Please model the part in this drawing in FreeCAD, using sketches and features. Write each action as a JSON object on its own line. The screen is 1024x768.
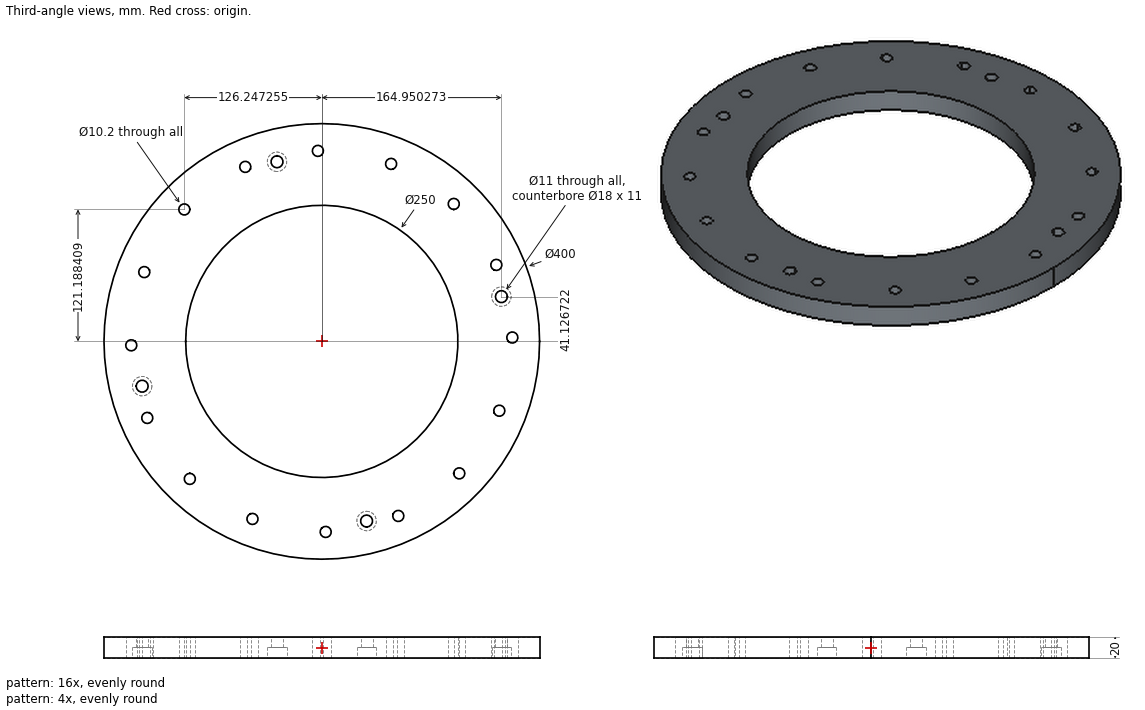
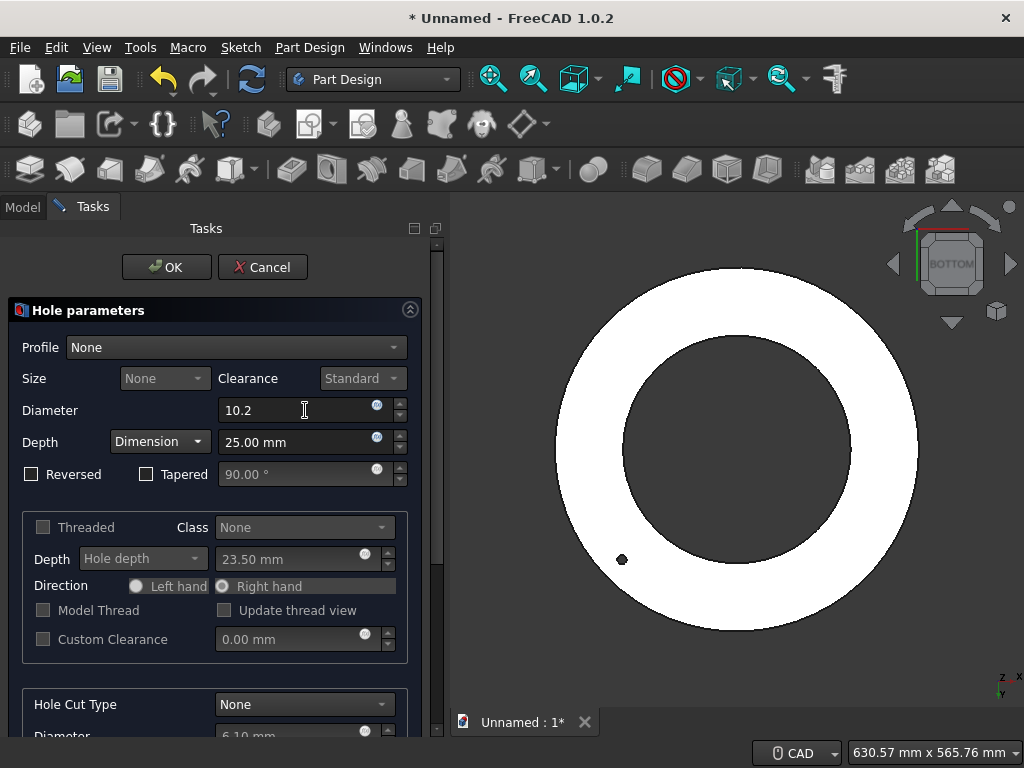
{"action": "left_click", "coordinate": [161, 442]}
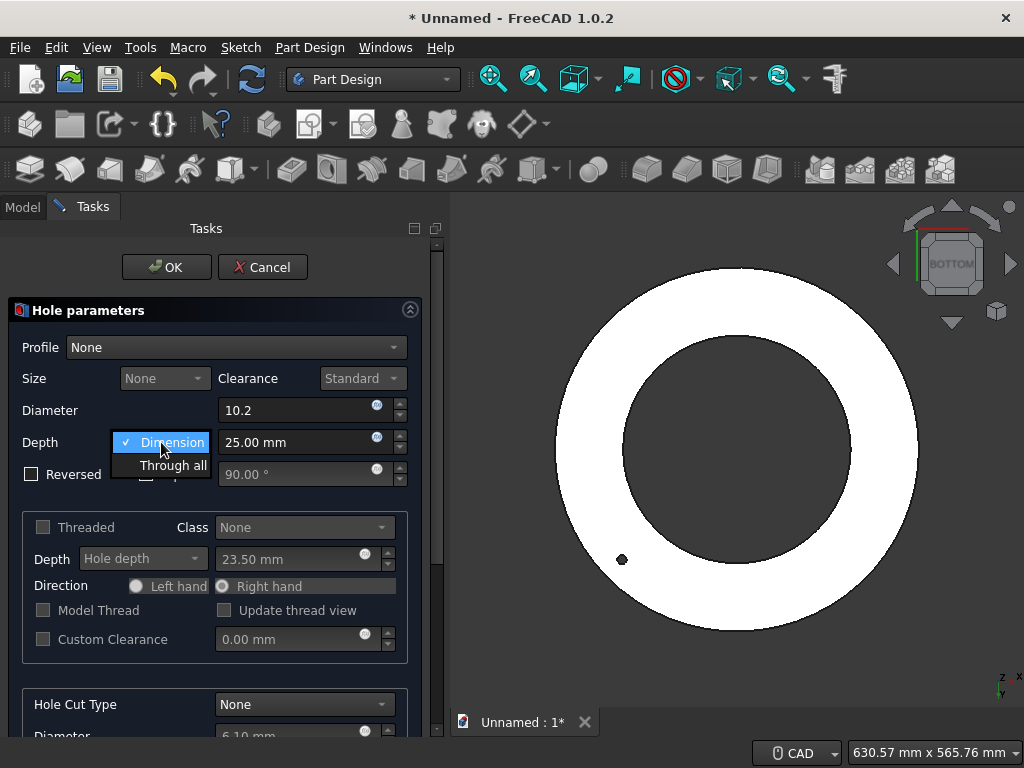
{"action": "left_click", "coordinate": [160, 466]}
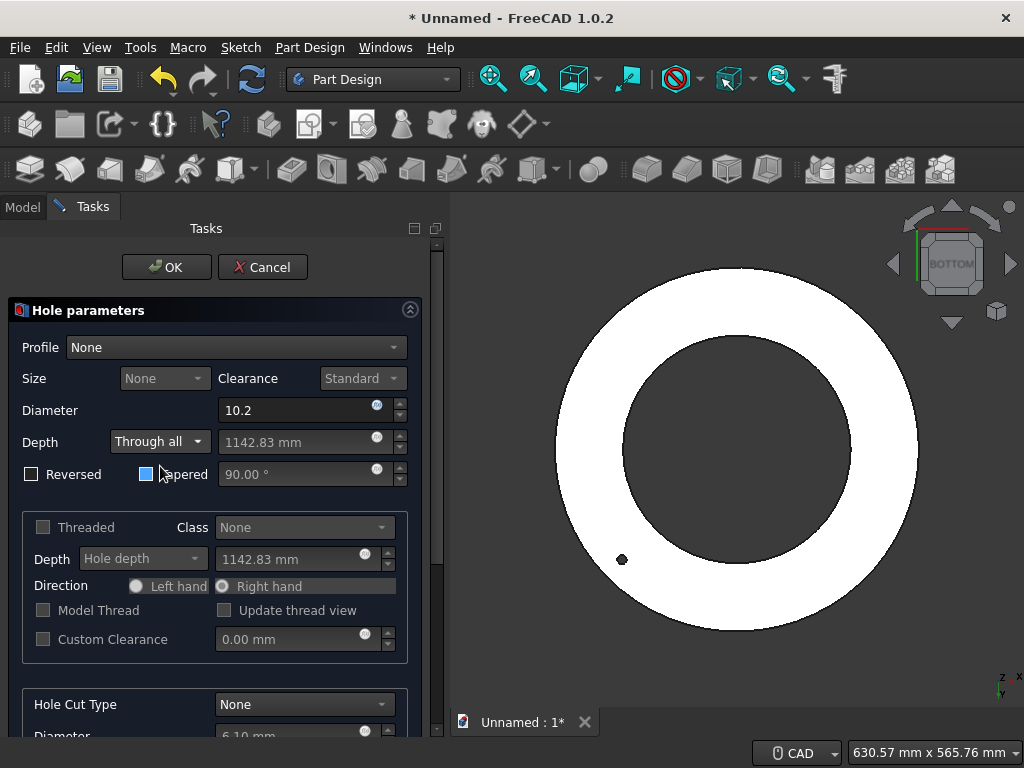
{"action": "left_click", "coordinate": [167, 267]}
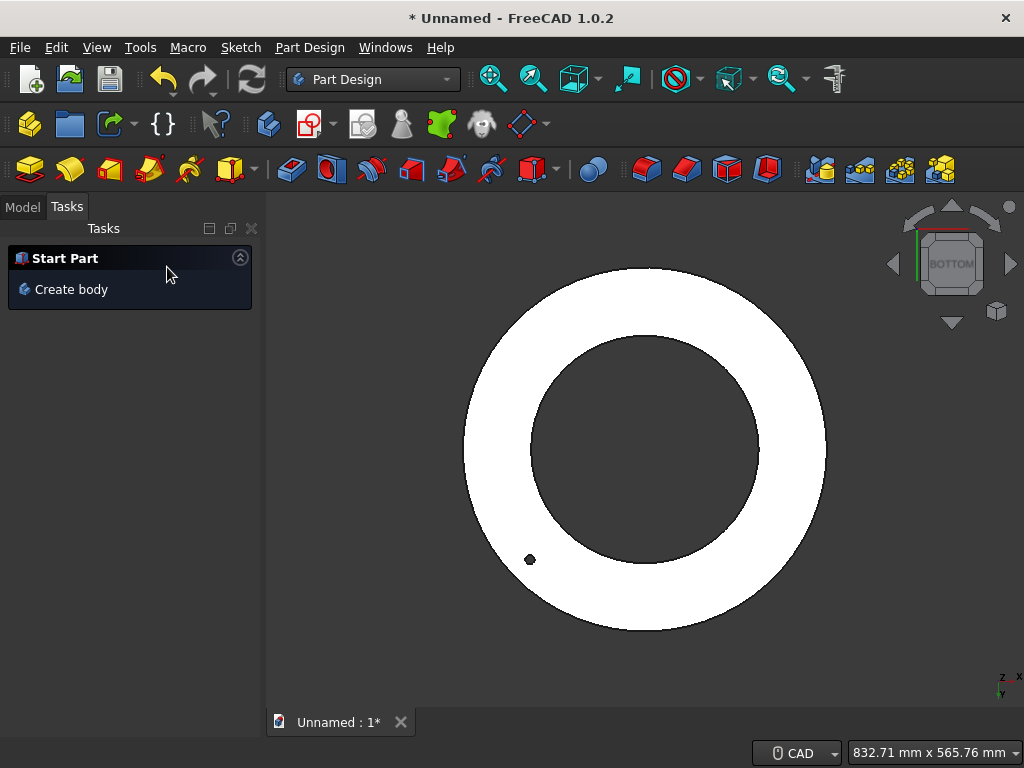
{"action": "left_click", "coordinate": [23, 206]}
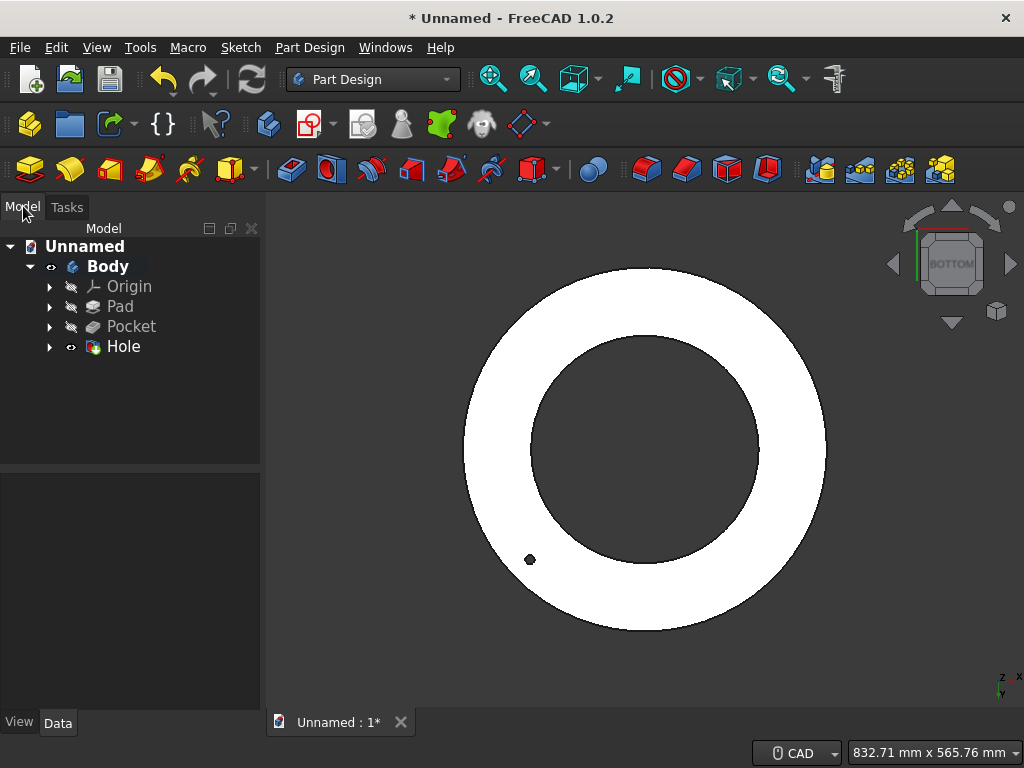
{"action": "left_click", "coordinate": [116, 347]}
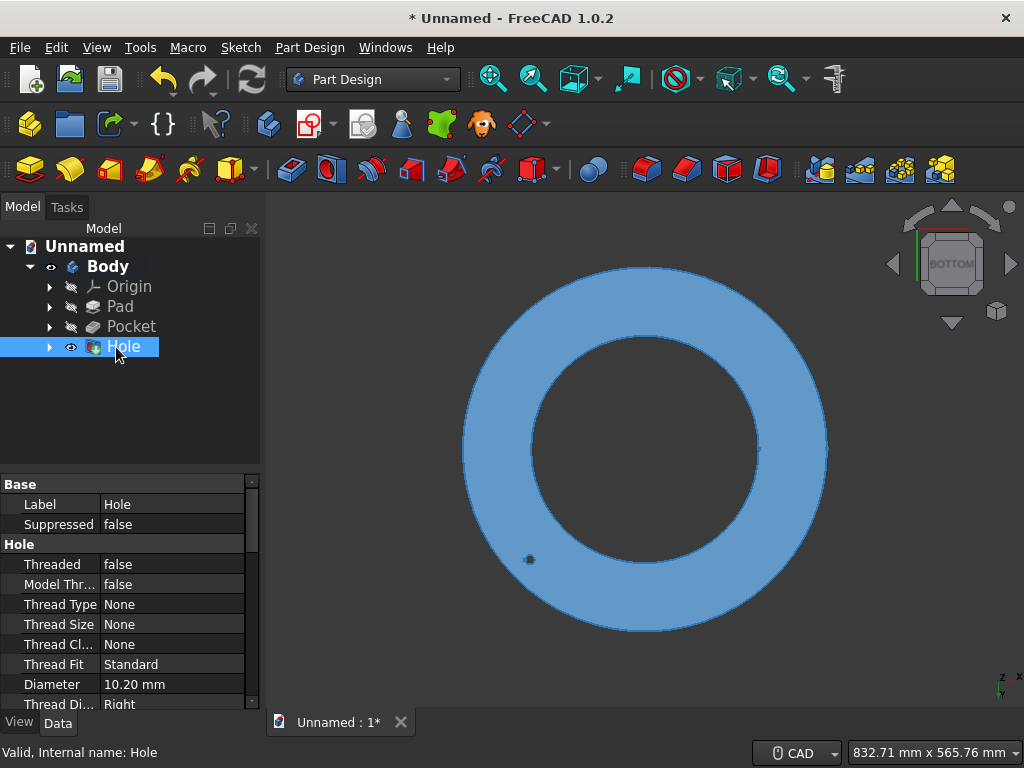
{"action": "left_click", "coordinate": [900, 170]}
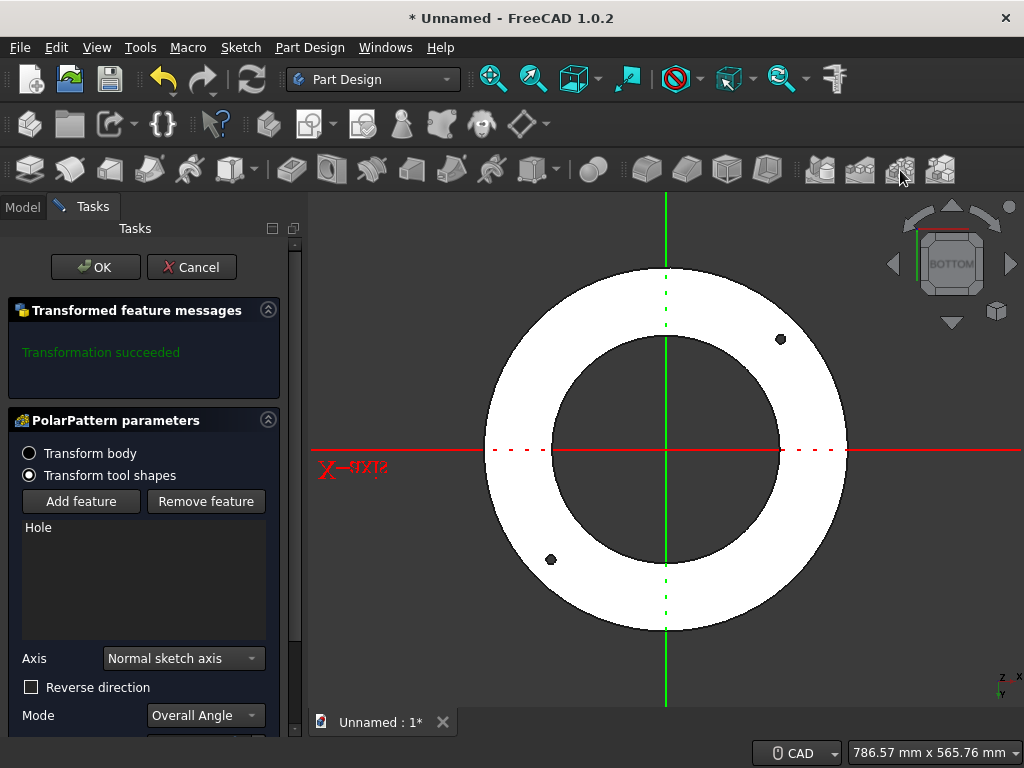
{"action": "left_click", "coordinate": [184, 658]}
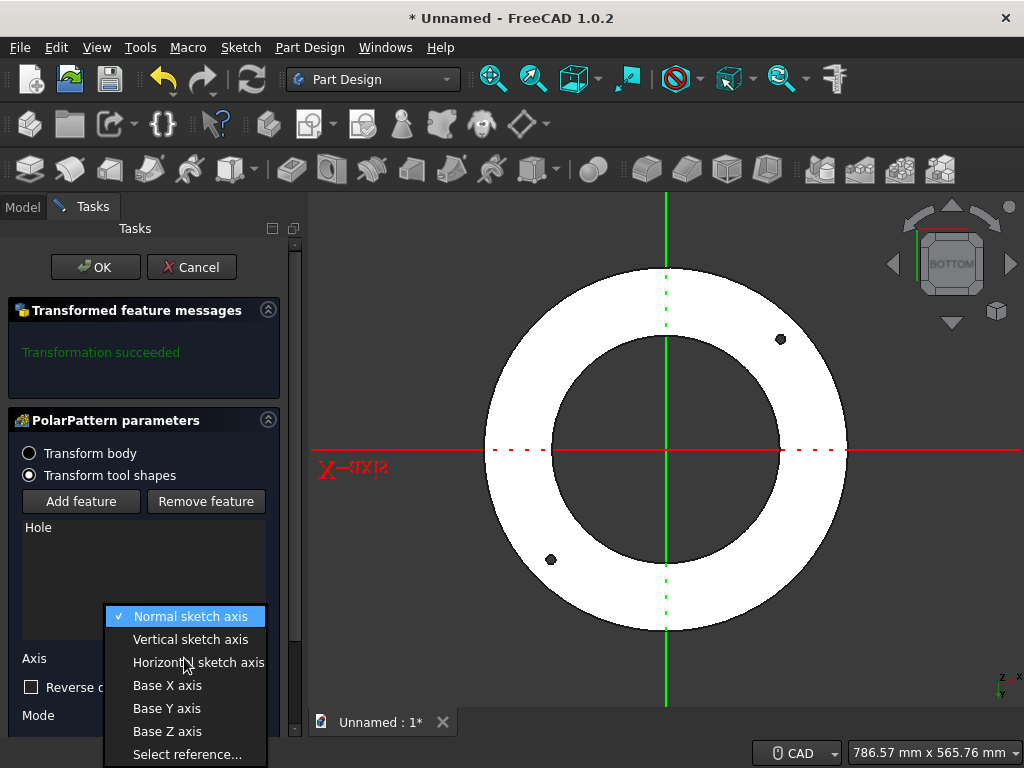
{"action": "left_click", "coordinate": [184, 732]}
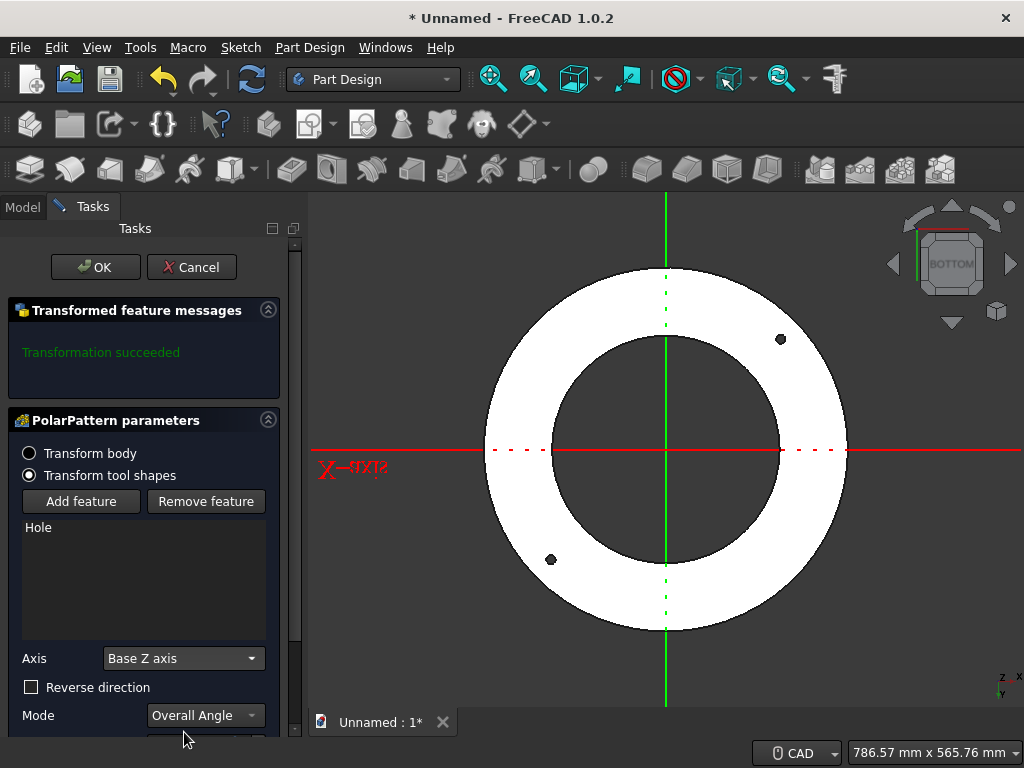
{"action": "scroll", "coordinate": [295, 487], "scroll_direction": "down", "scroll_amount": 2}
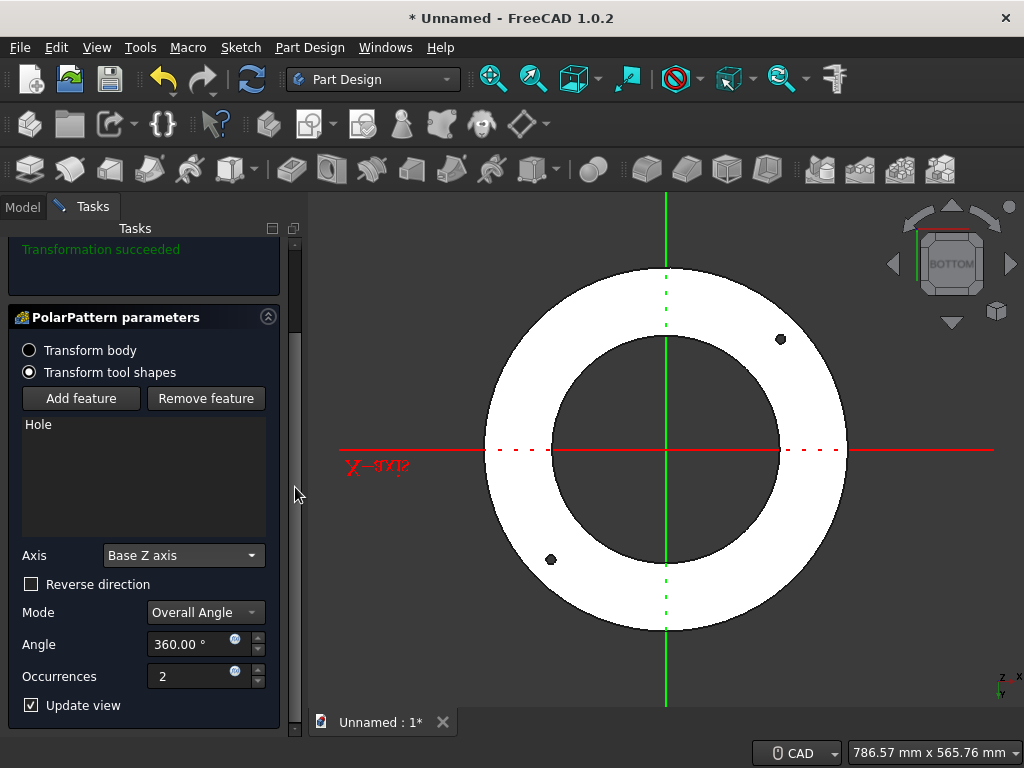
{"action": "triple_click", "coordinate": [198, 676]}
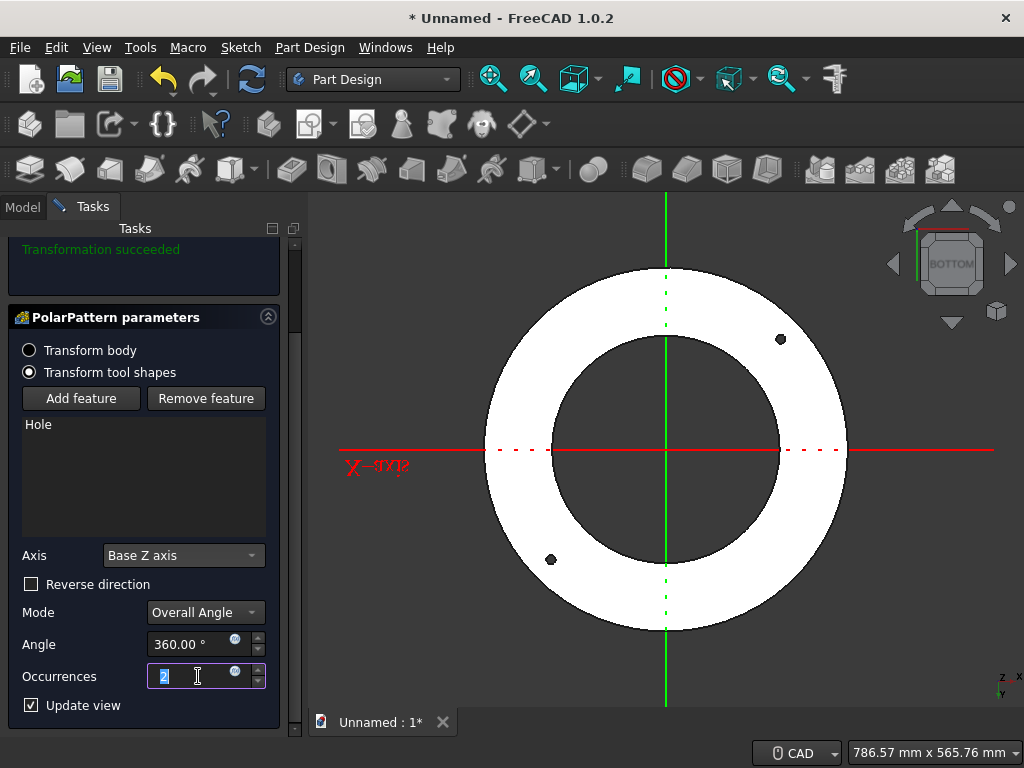
{"action": "type", "text": "16"}
{"action": "key", "text": "Tab"}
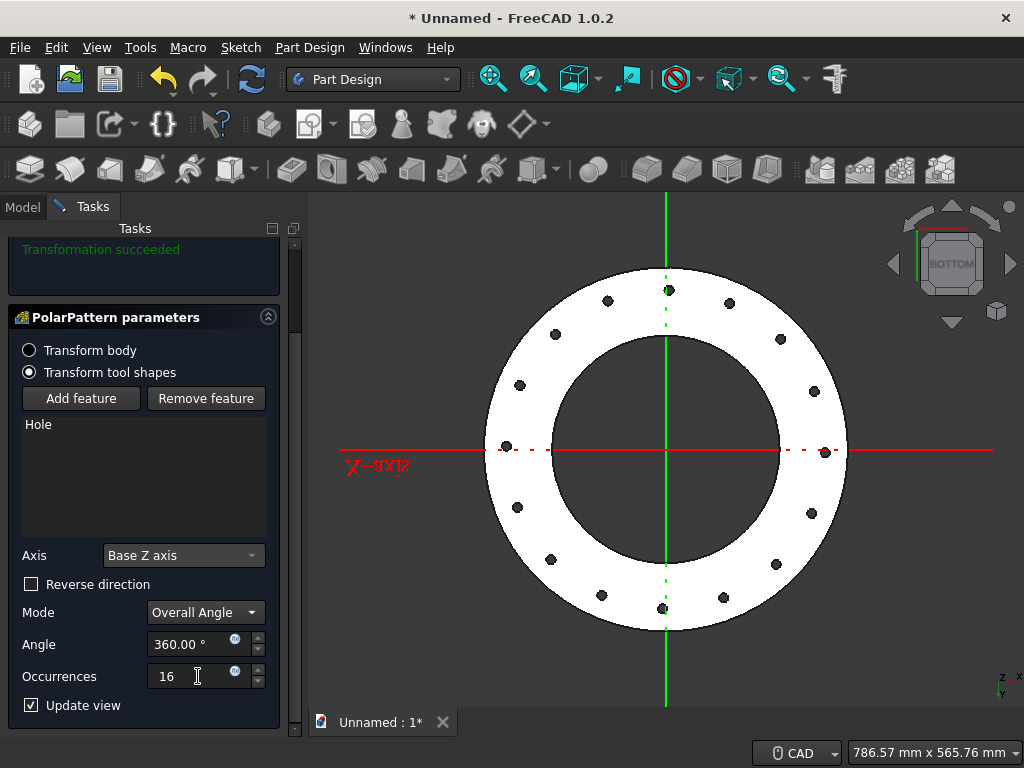
{"action": "scroll", "coordinate": [295, 487], "scroll_direction": "up", "scroll_amount": 3}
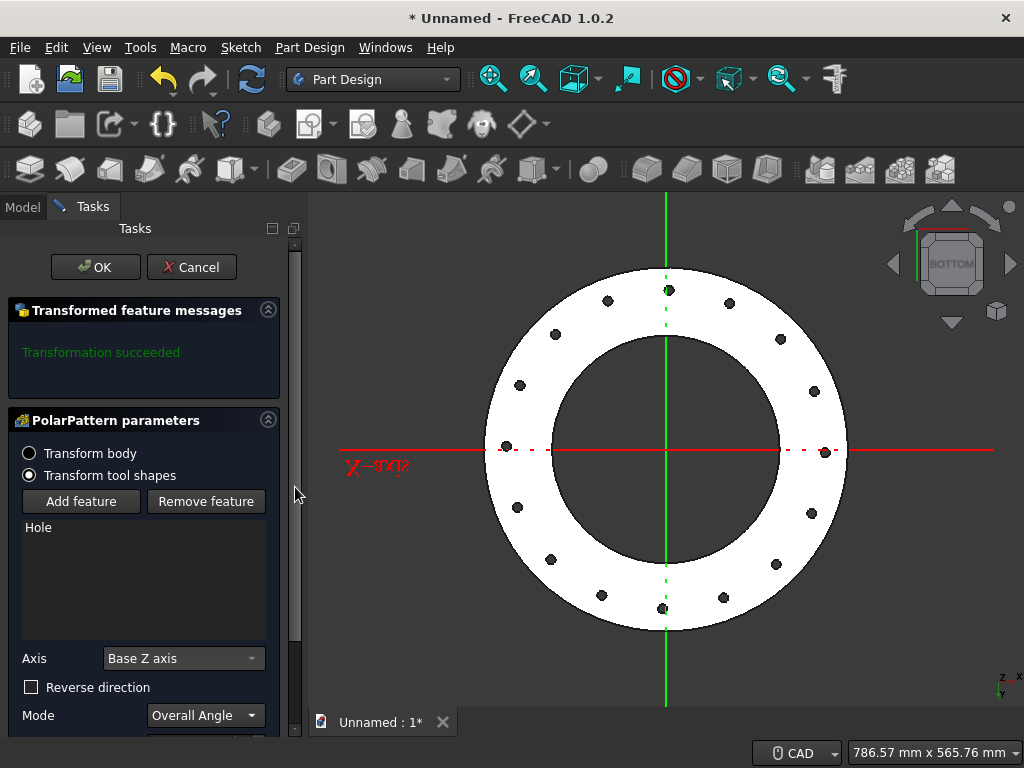
{"action": "left_click", "coordinate": [96, 267]}